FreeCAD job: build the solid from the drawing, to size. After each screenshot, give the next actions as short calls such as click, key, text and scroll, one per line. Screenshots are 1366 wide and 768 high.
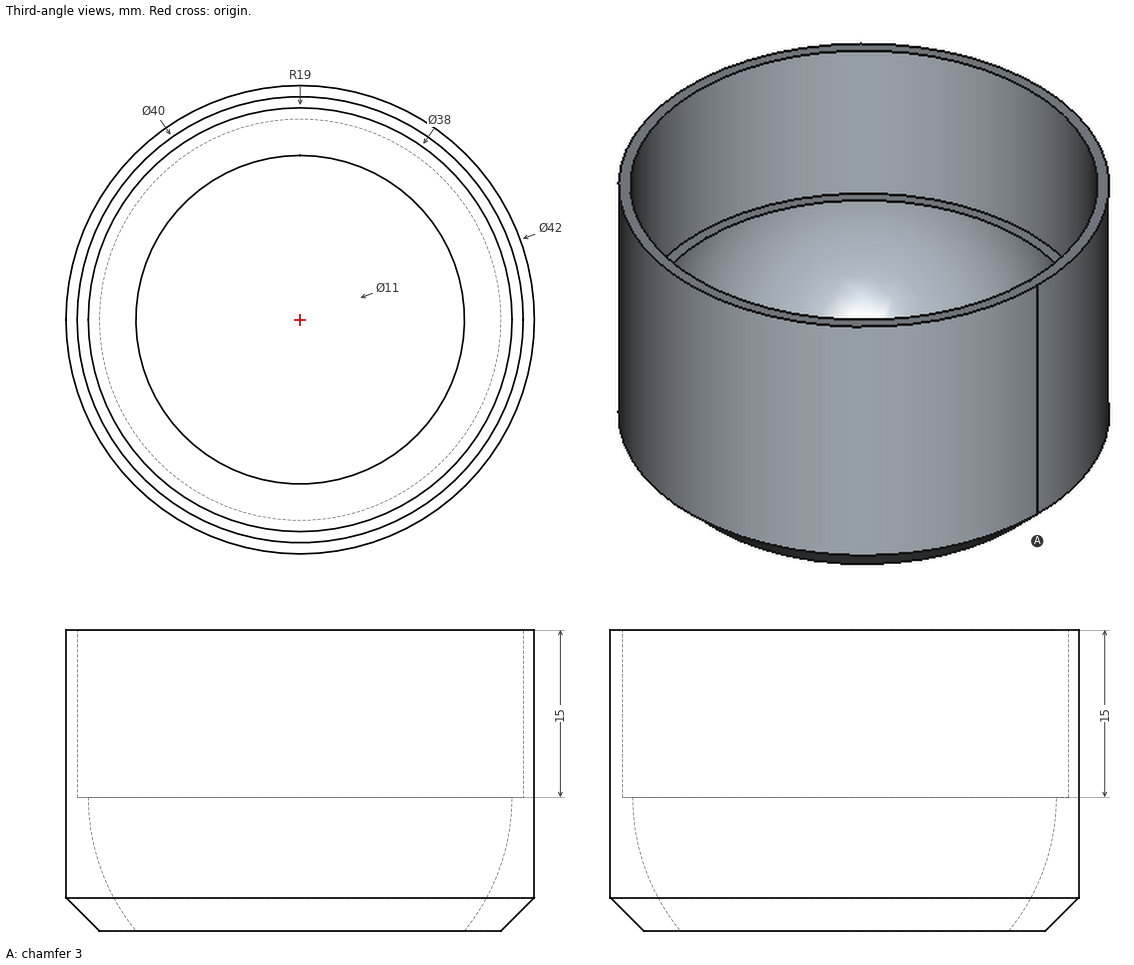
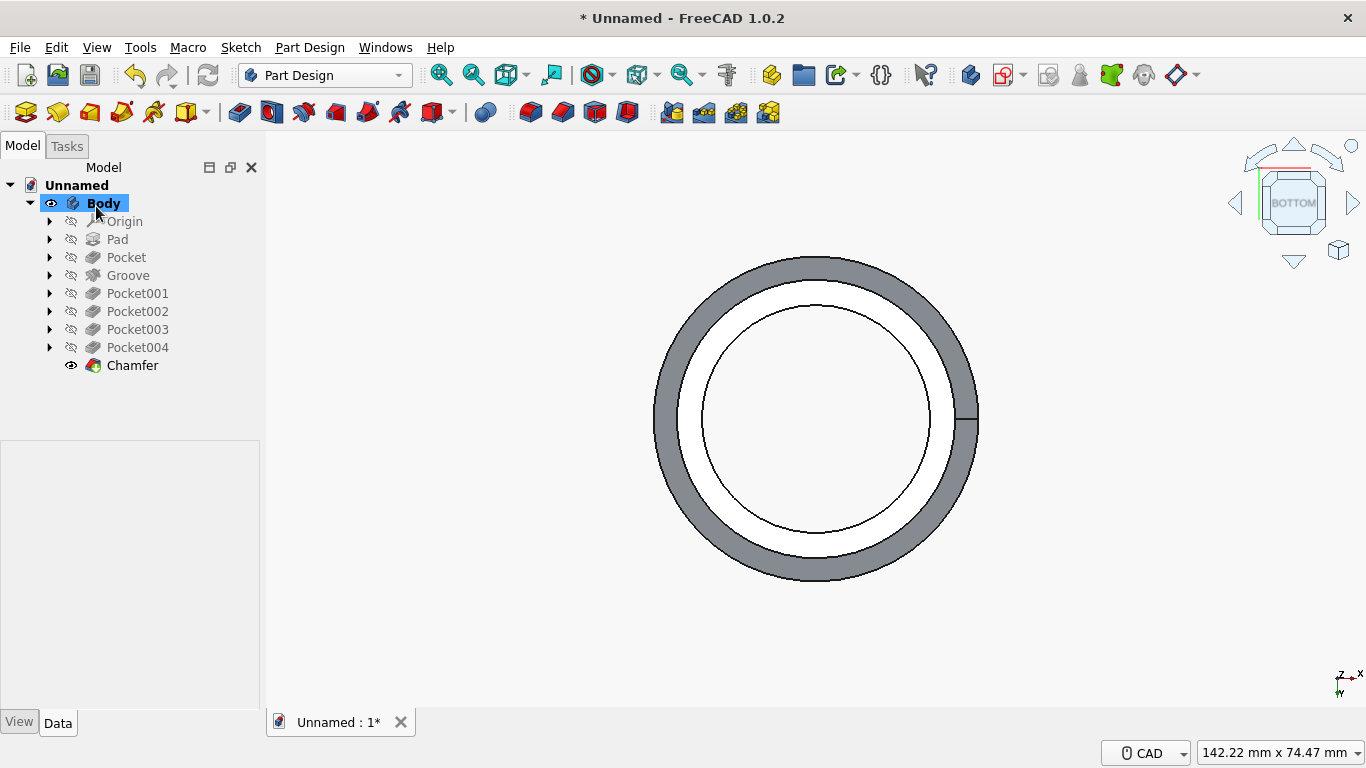
key(0)